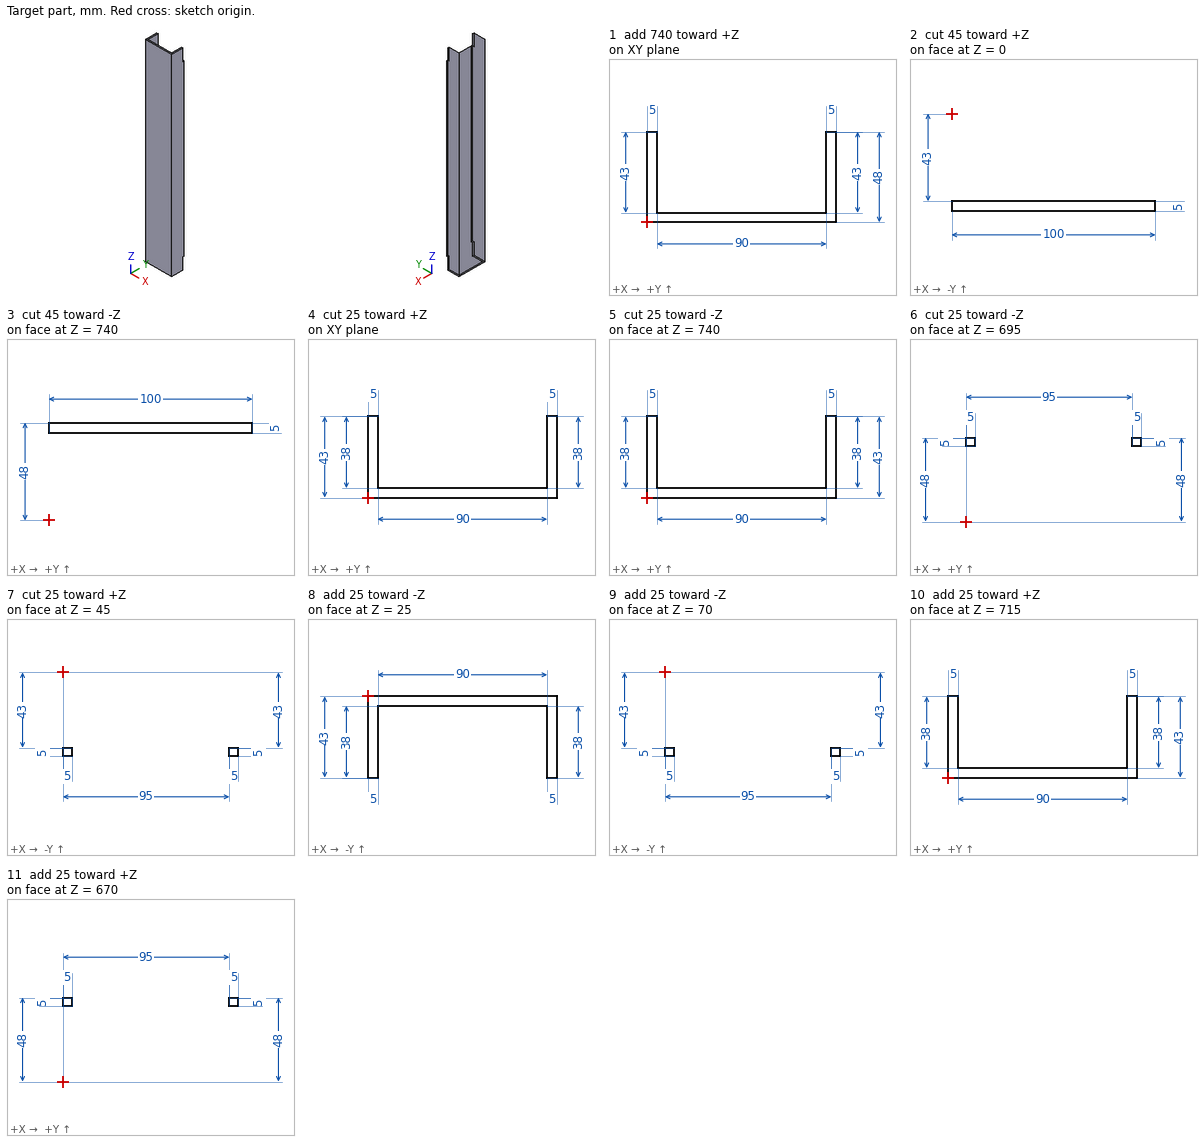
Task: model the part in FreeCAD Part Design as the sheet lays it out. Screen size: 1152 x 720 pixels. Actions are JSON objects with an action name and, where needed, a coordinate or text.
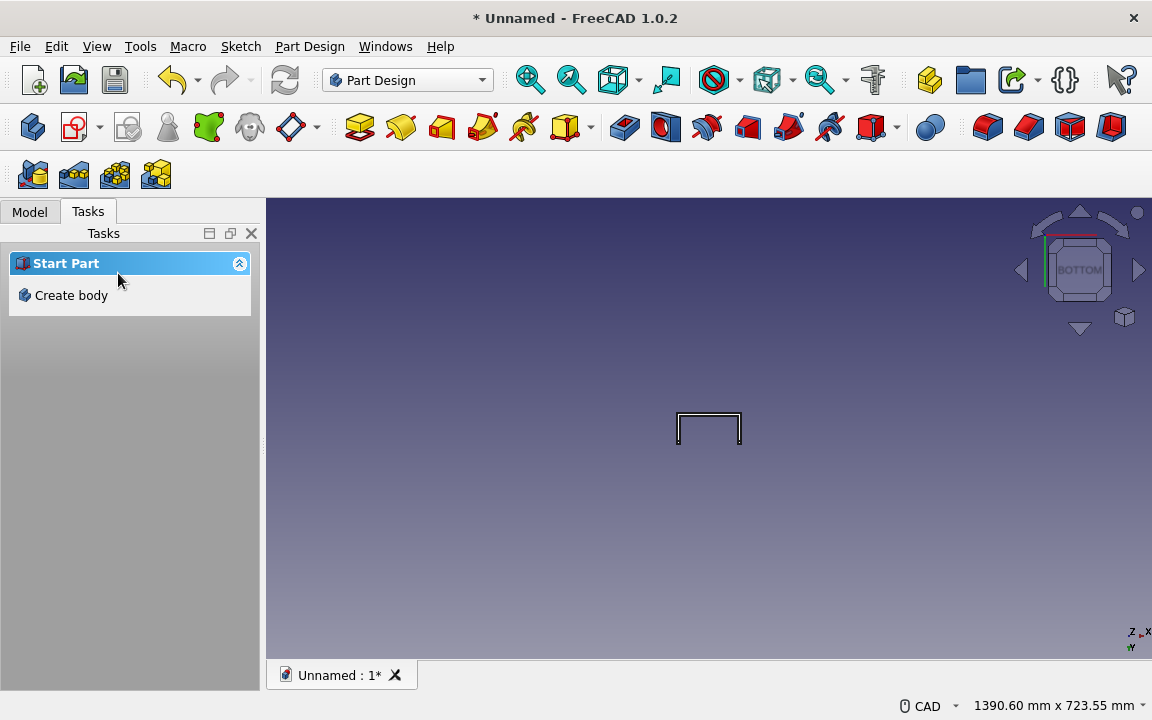
{"action": "key", "text": "0"}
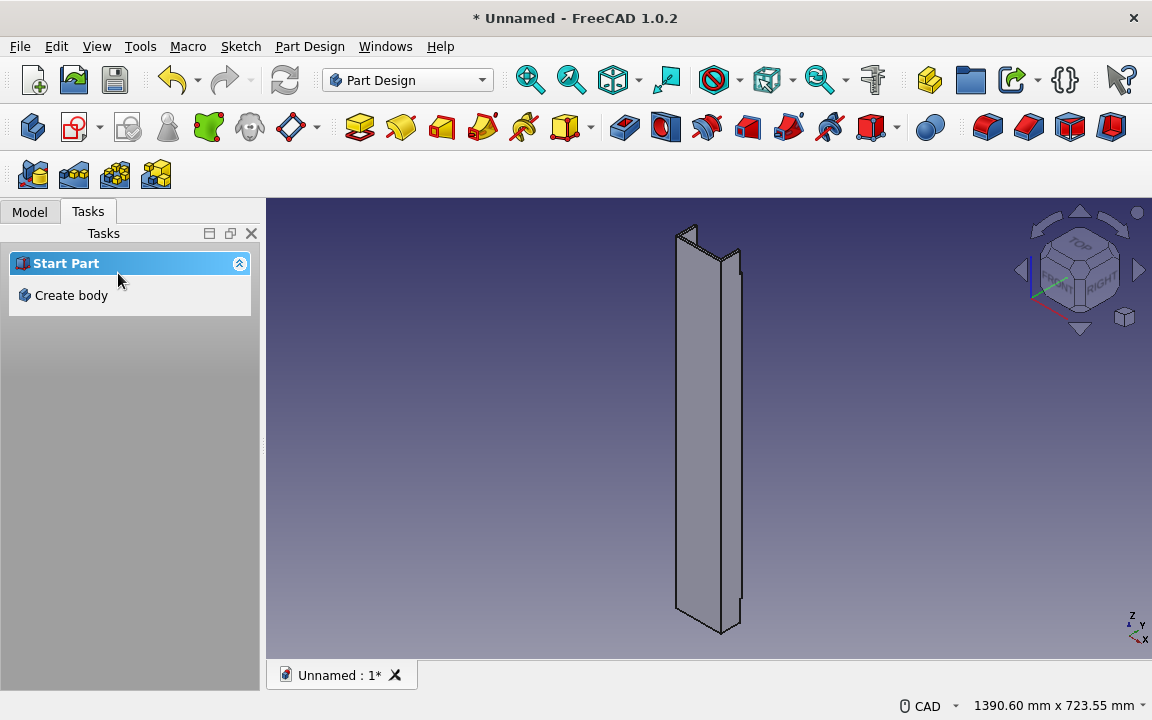
{"action": "scroll", "coordinate": [719, 258], "scroll_direction": "up", "scroll_amount": 12}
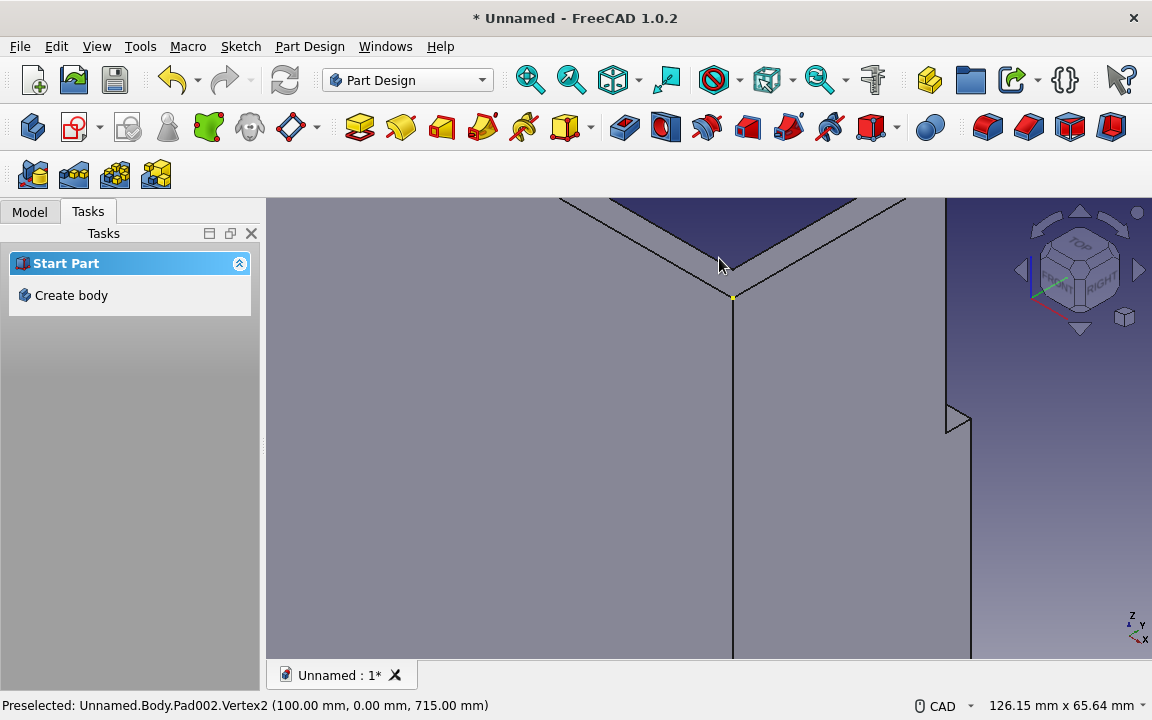
{"action": "left_click", "coordinate": [713, 268]}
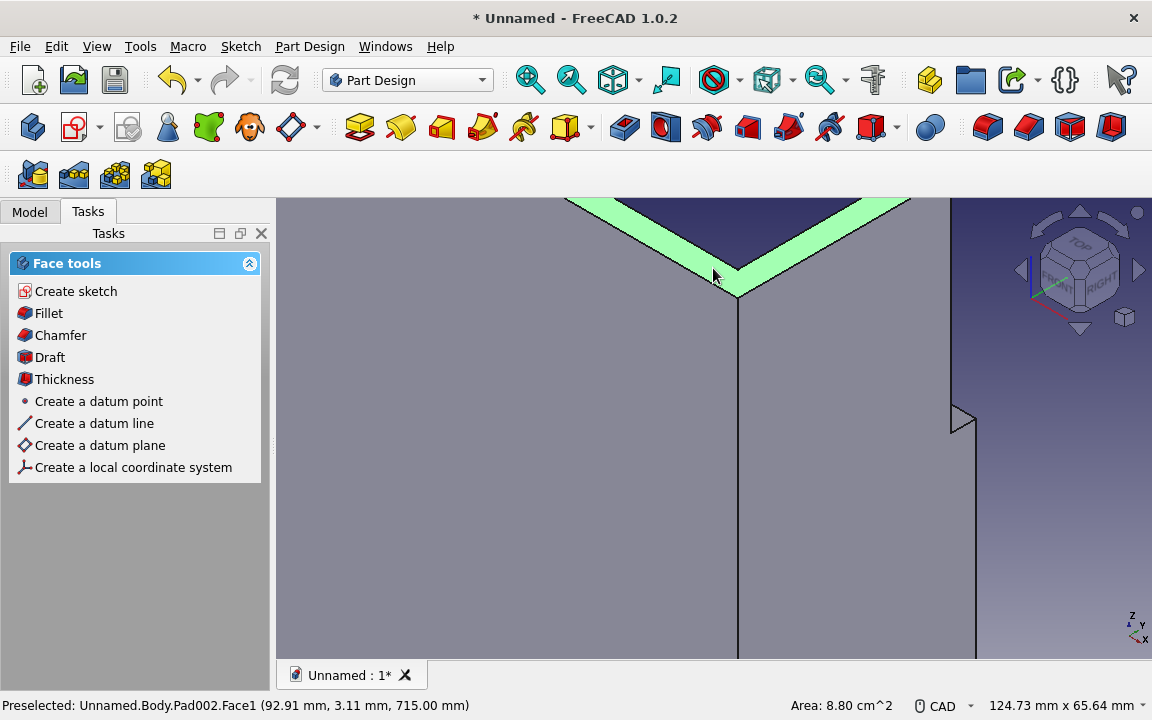
{"action": "left_click", "coordinate": [74, 128]}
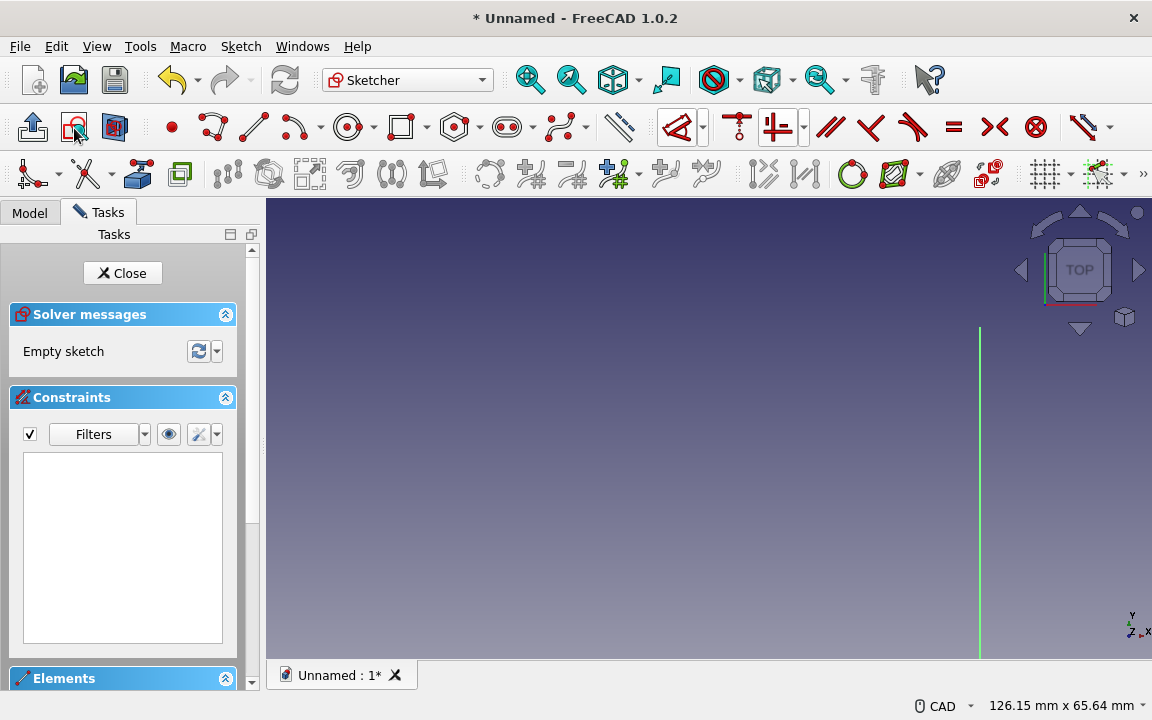
{"action": "scroll", "coordinate": [640, 428], "scroll_direction": "down", "scroll_amount": 5}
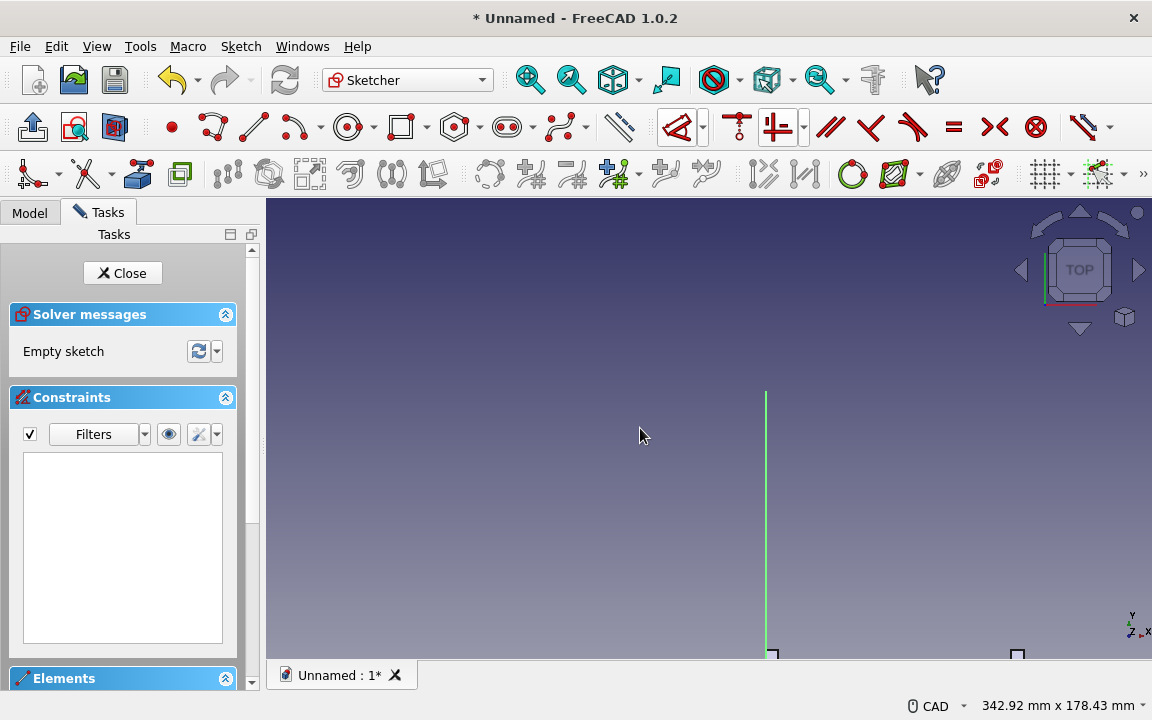
{"action": "scroll", "coordinate": [640, 428], "scroll_direction": "down", "scroll_amount": 5}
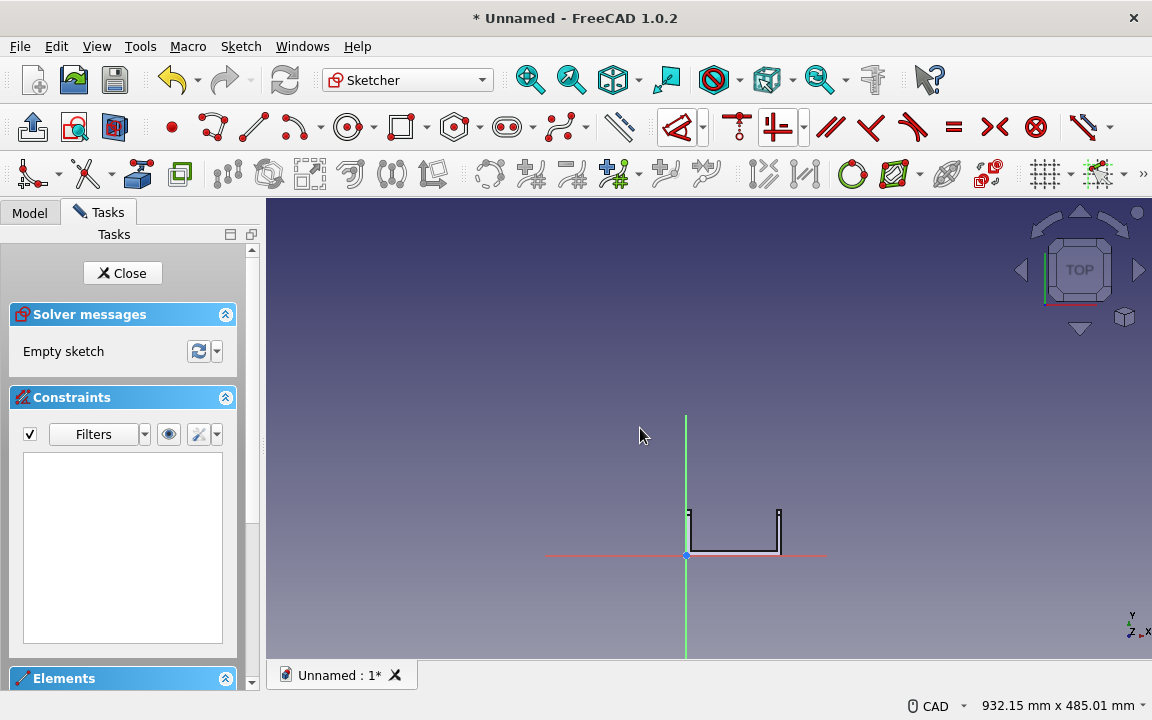
{"action": "scroll", "coordinate": [758, 562], "scroll_direction": "up", "scroll_amount": 8}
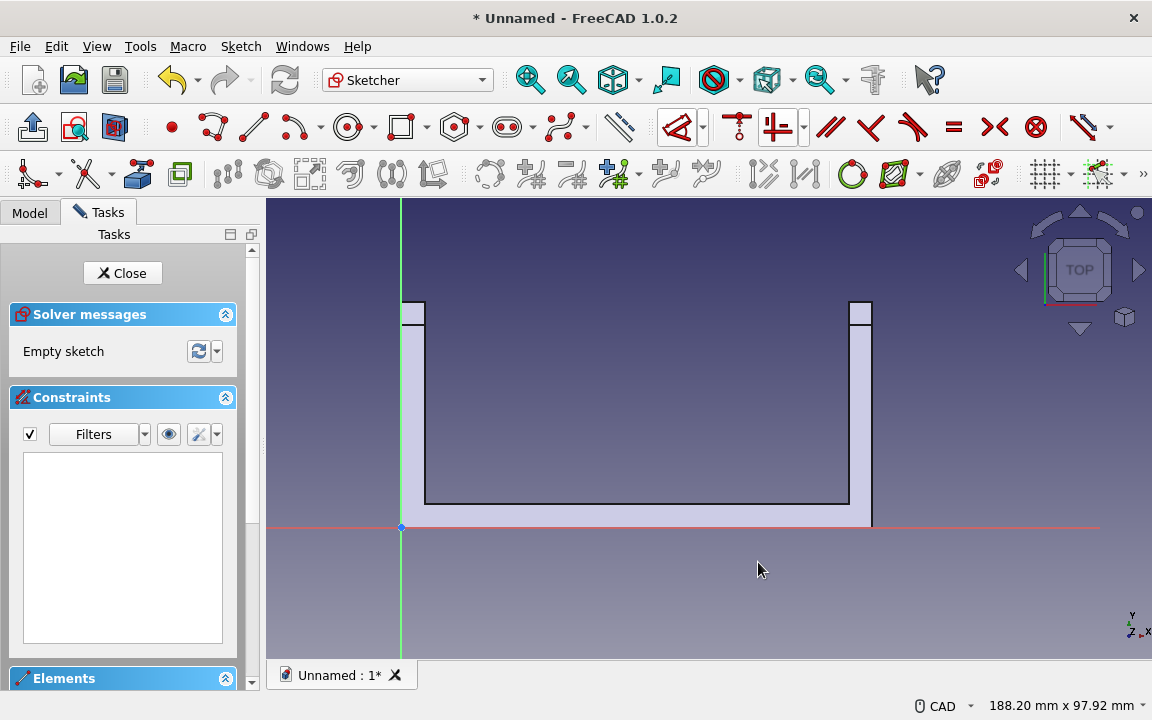
{"action": "left_click", "coordinate": [213, 128]}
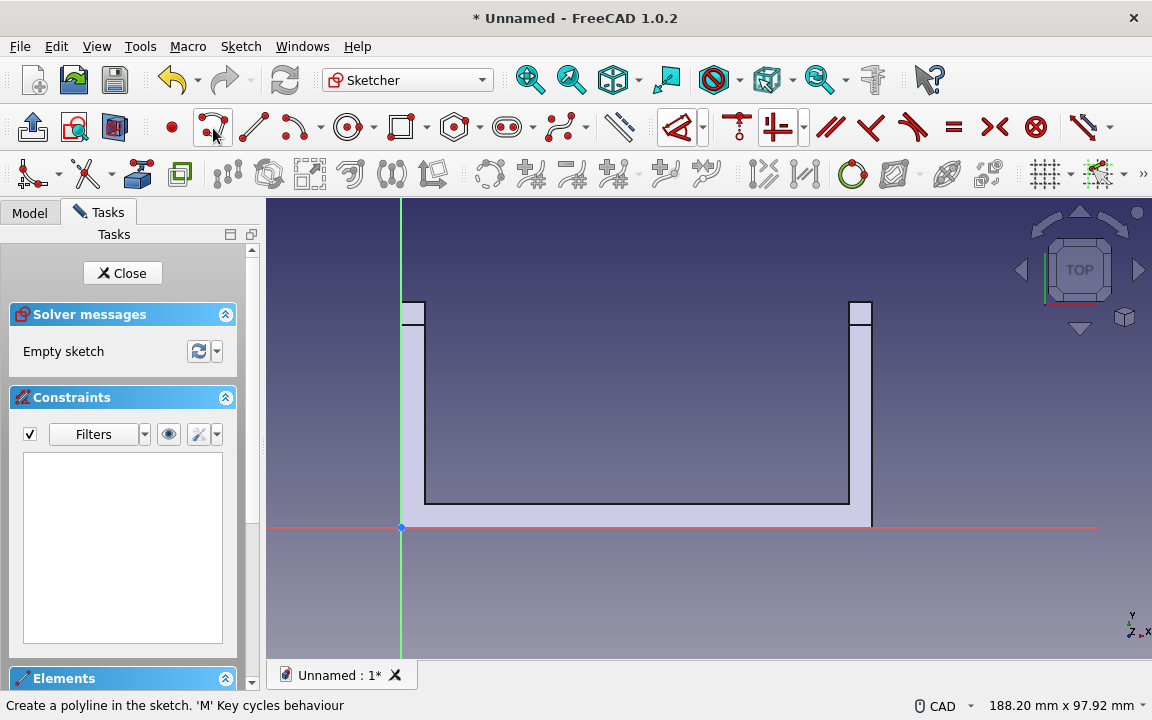
{"action": "left_click", "coordinate": [401, 528]}
{"action": "left_click", "coordinate": [872, 519]}
{"action": "left_click", "coordinate": [872, 325]}
{"action": "left_click", "coordinate": [849, 325]}
{"action": "left_click", "coordinate": [849, 504]}
{"action": "left_click", "coordinate": [425, 504]}
{"action": "left_click", "coordinate": [425, 325]}
{"action": "left_click", "coordinate": [410, 325]}
{"action": "left_click", "coordinate": [401, 528]}
{"action": "key", "text": "Escape"}
{"action": "key", "text": "Escape"}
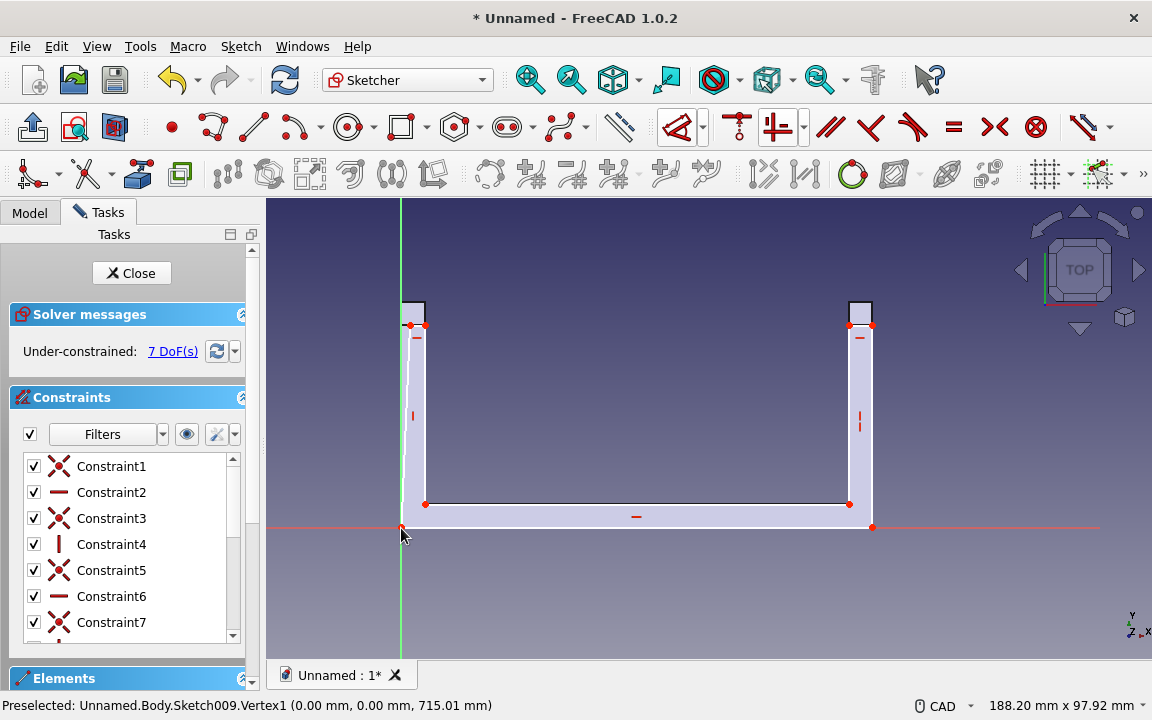
{"action": "left_click", "coordinate": [404, 467]}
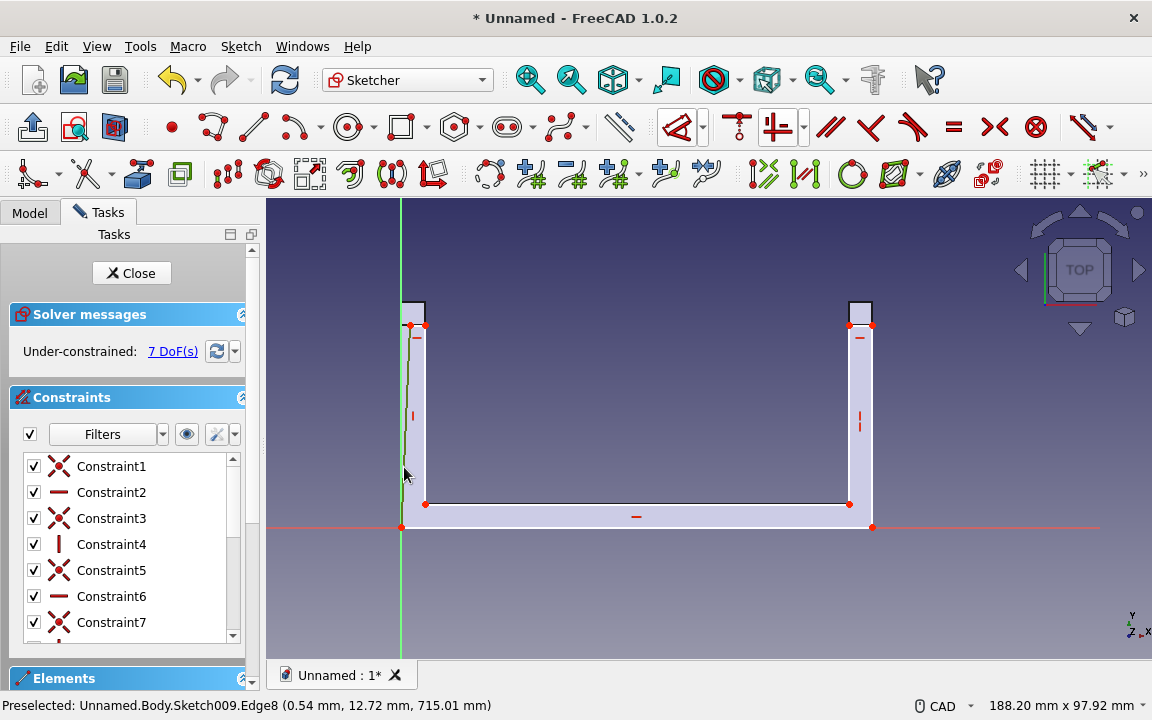
{"action": "left_click", "coordinate": [804, 128]}